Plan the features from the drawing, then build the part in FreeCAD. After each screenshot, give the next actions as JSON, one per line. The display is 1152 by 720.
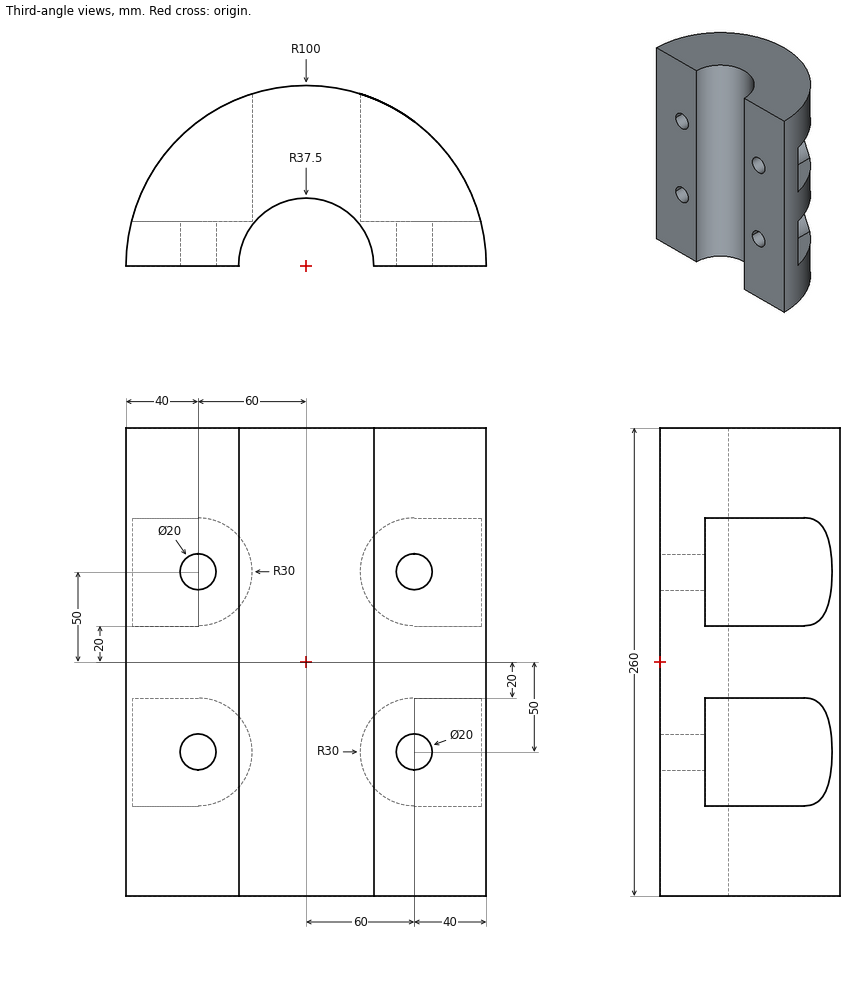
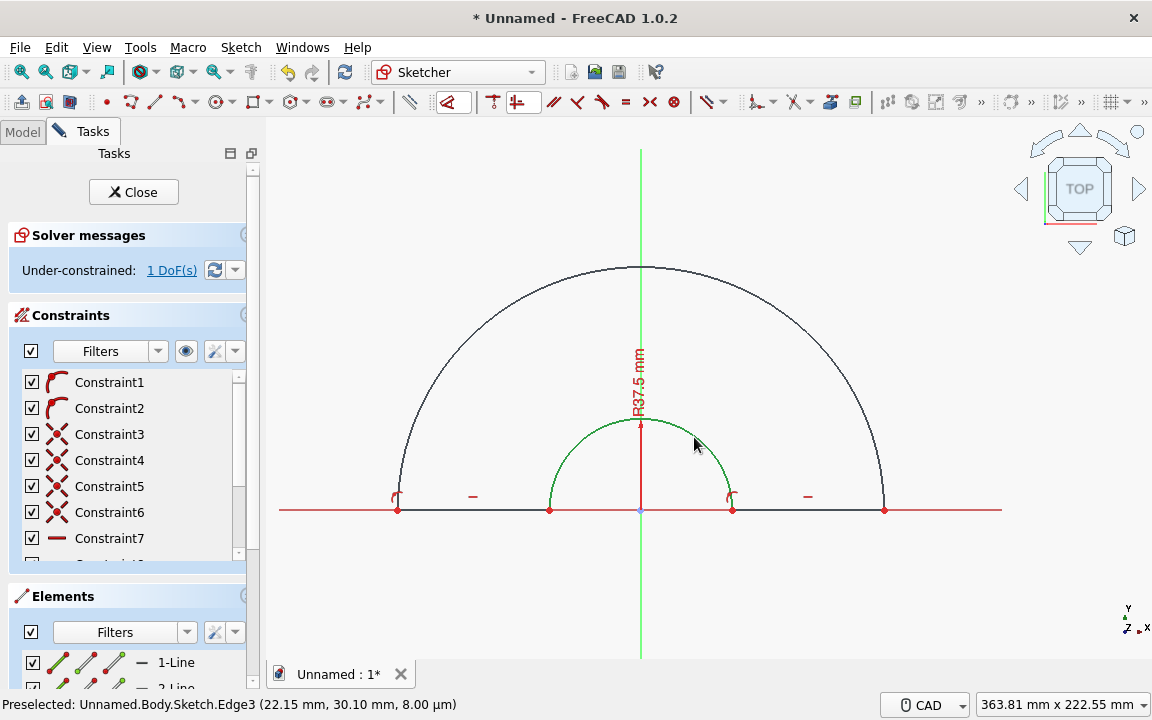
{"action": "left_click", "coordinate": [784, 313]}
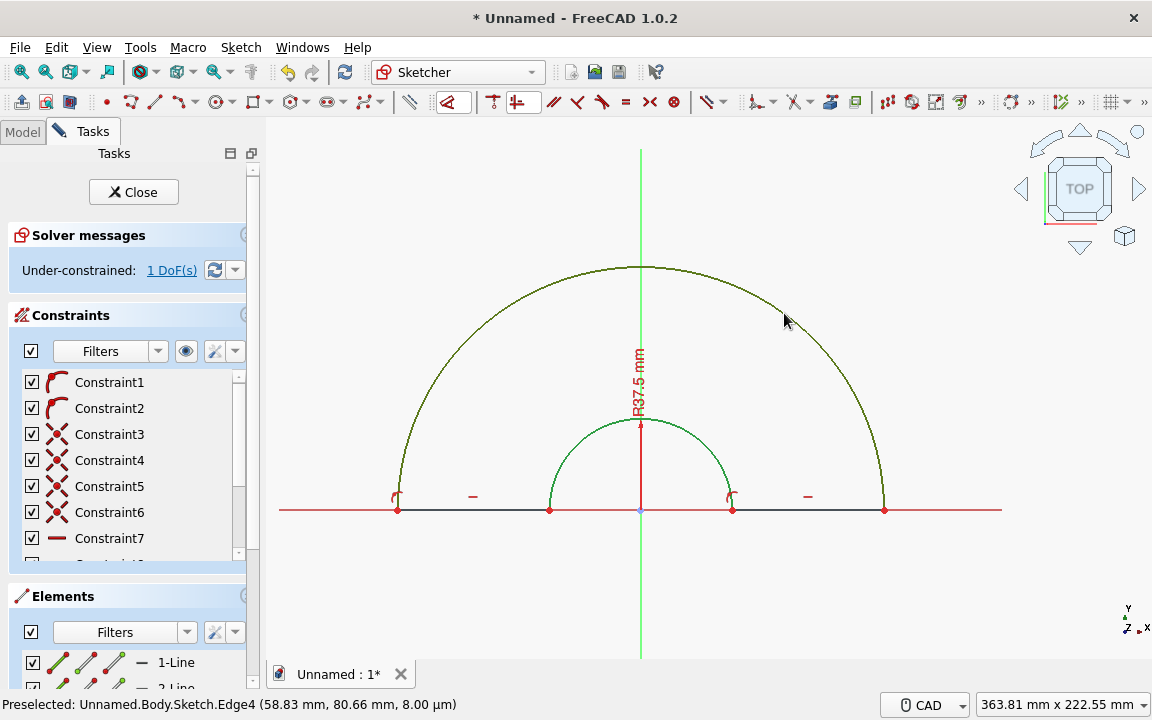
{"action": "key", "text": "k r"}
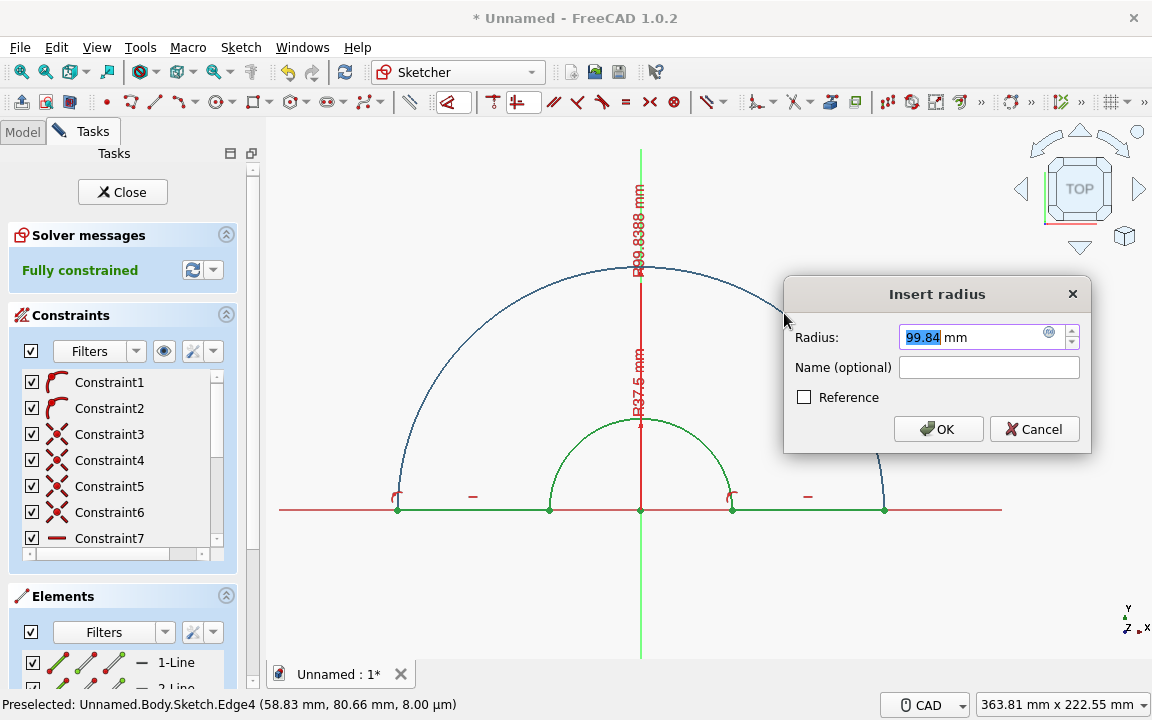
{"action": "type", "text": "100"}
{"action": "key", "text": "Return"}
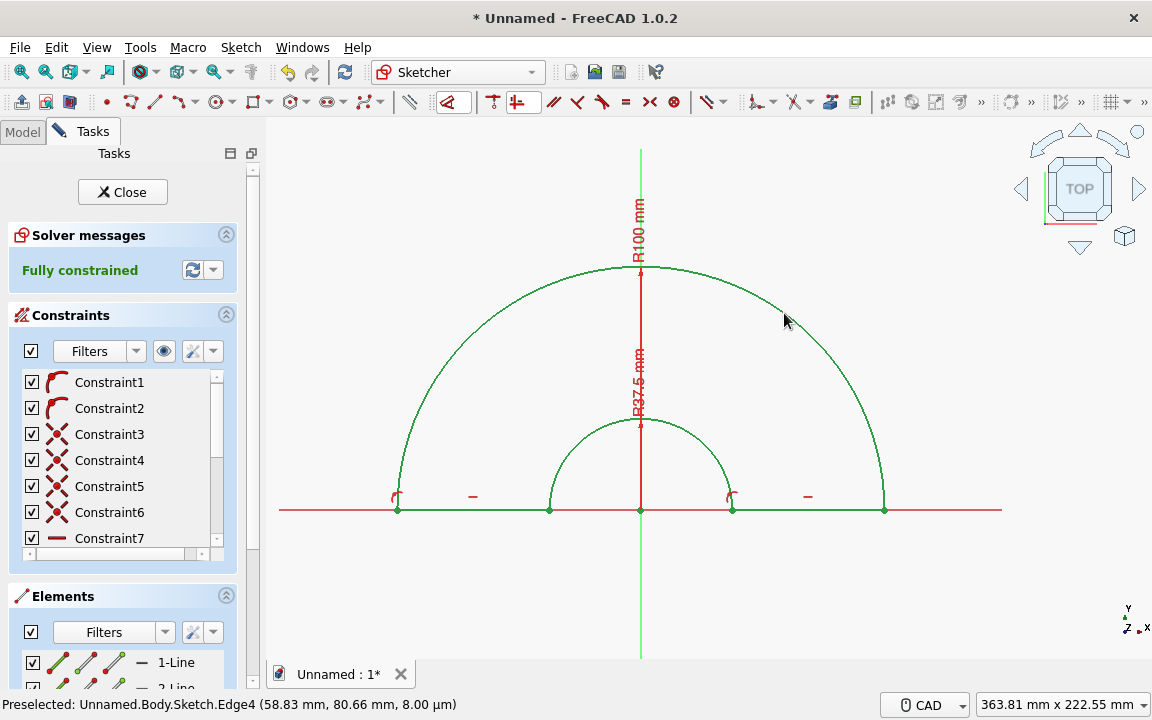
{"action": "left_click", "coordinate": [123, 192]}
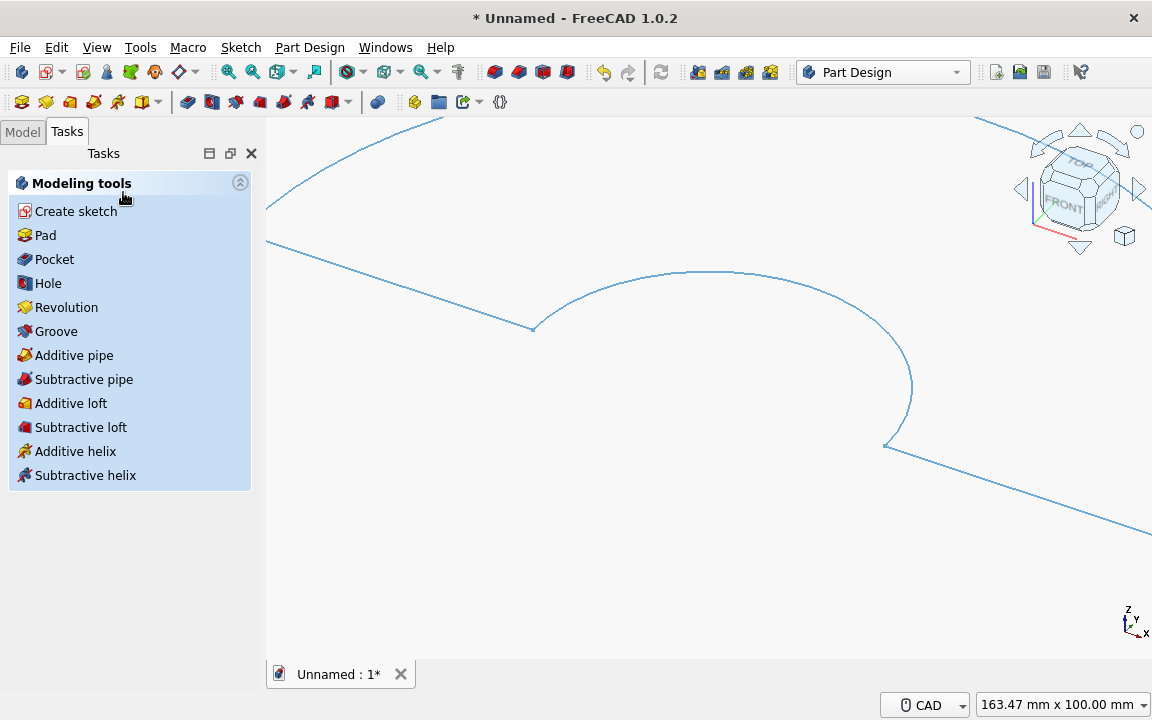
{"action": "left_click", "coordinate": [22, 102]}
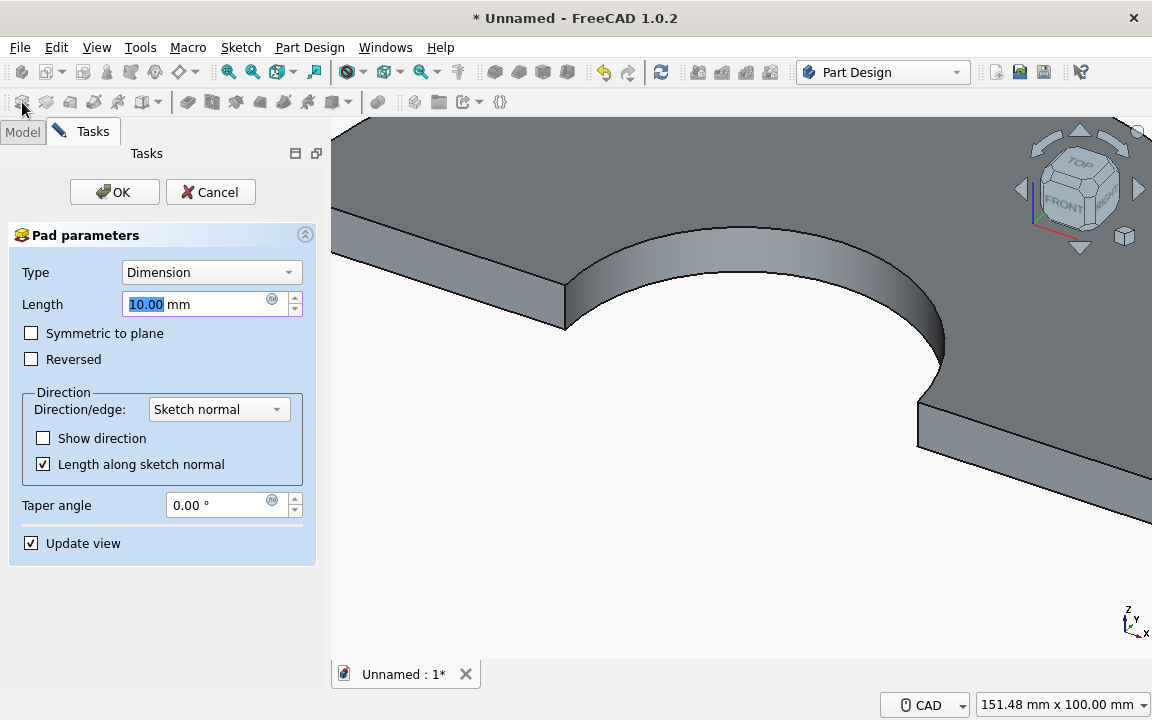
{"action": "type", "text": "260"}
{"action": "key", "text": "Tab"}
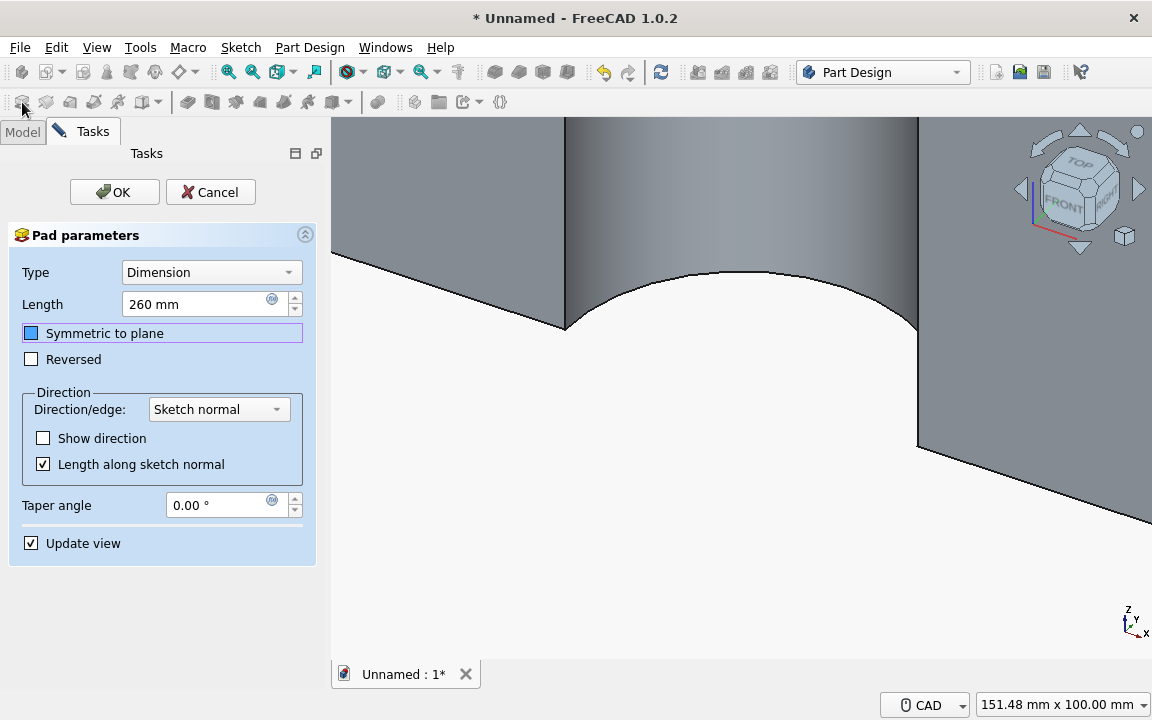
{"action": "left_click", "coordinate": [30, 333]}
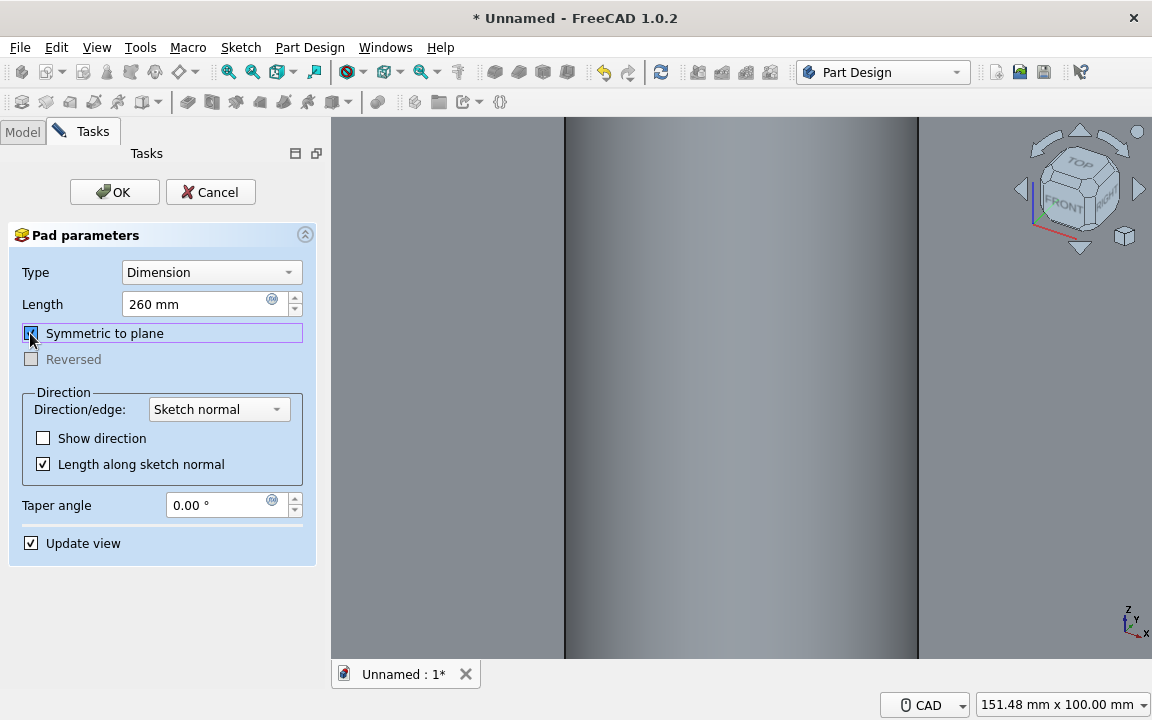
{"action": "left_click", "coordinate": [115, 192]}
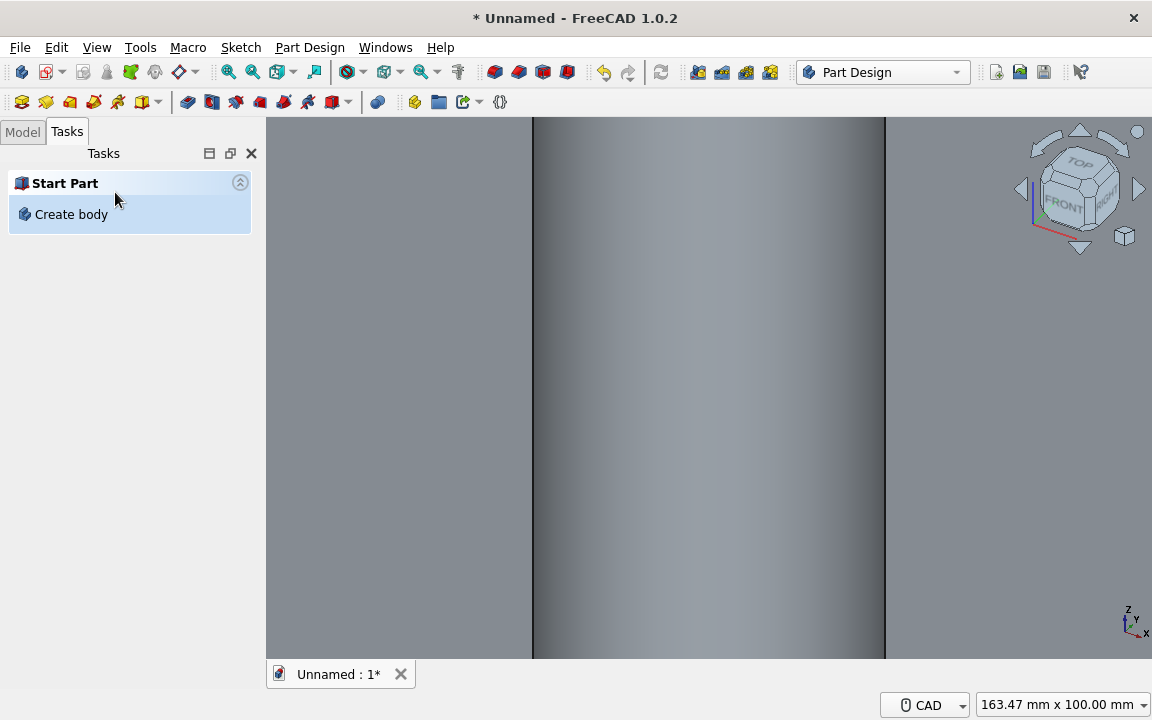
{"action": "left_click", "coordinate": [230, 72]}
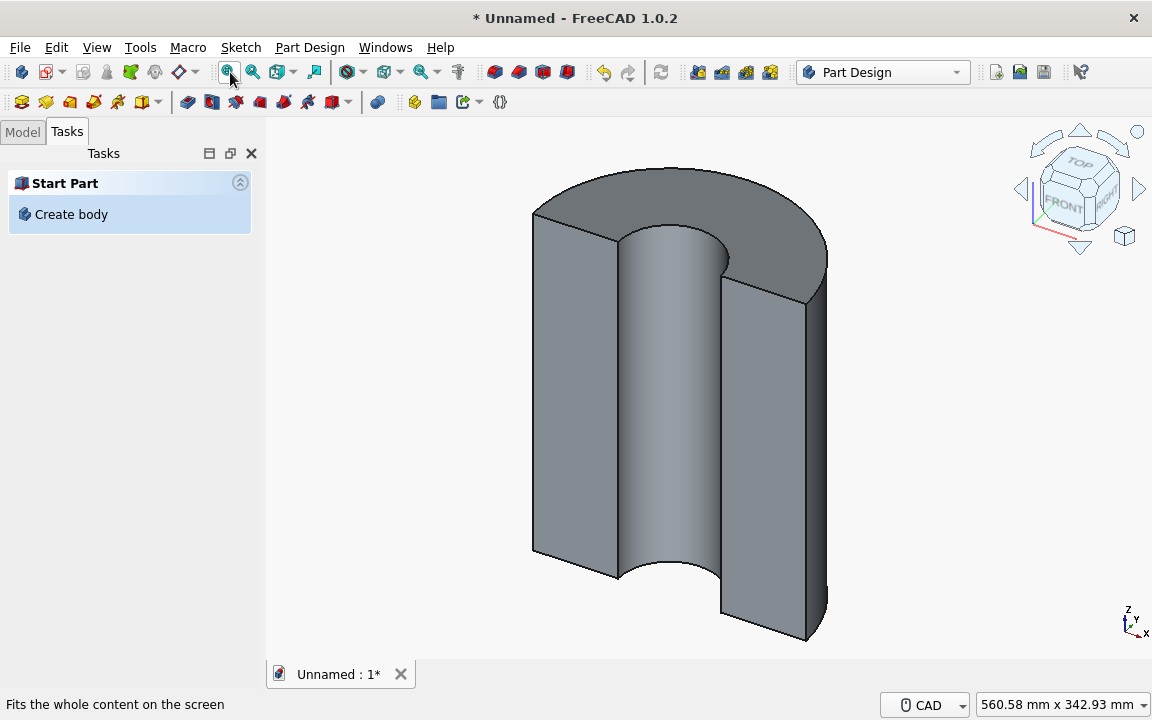
{"action": "left_click", "coordinate": [23, 131]}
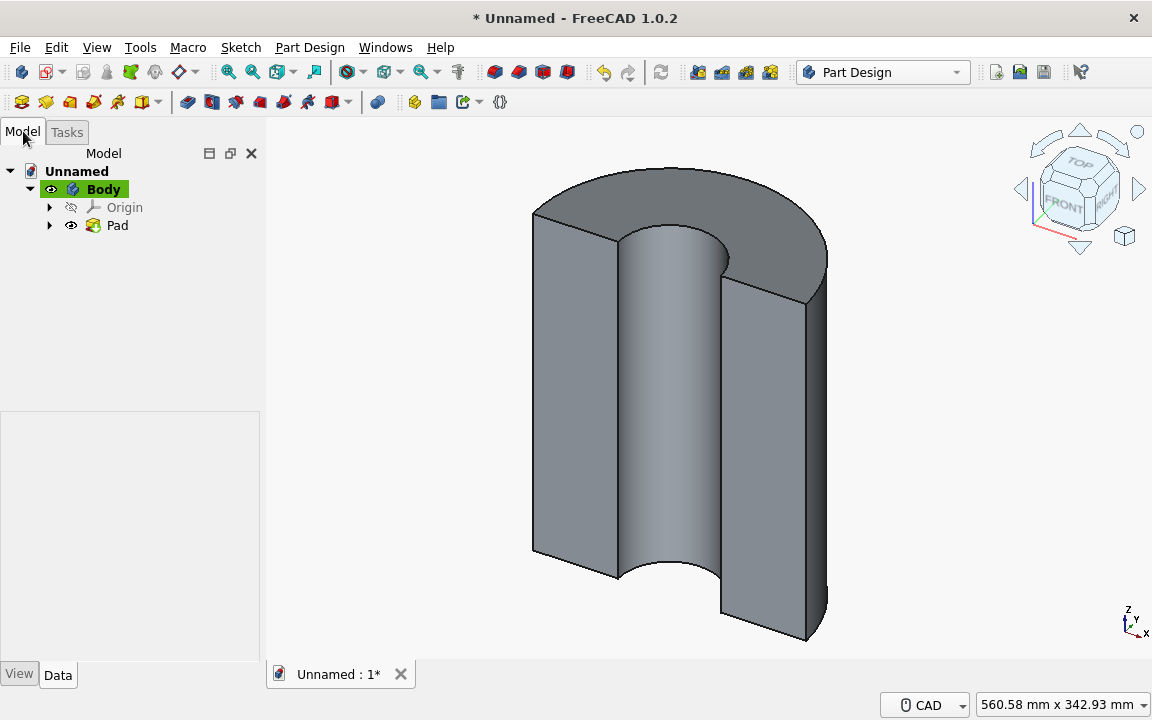
{"action": "left_click", "coordinate": [50, 207]}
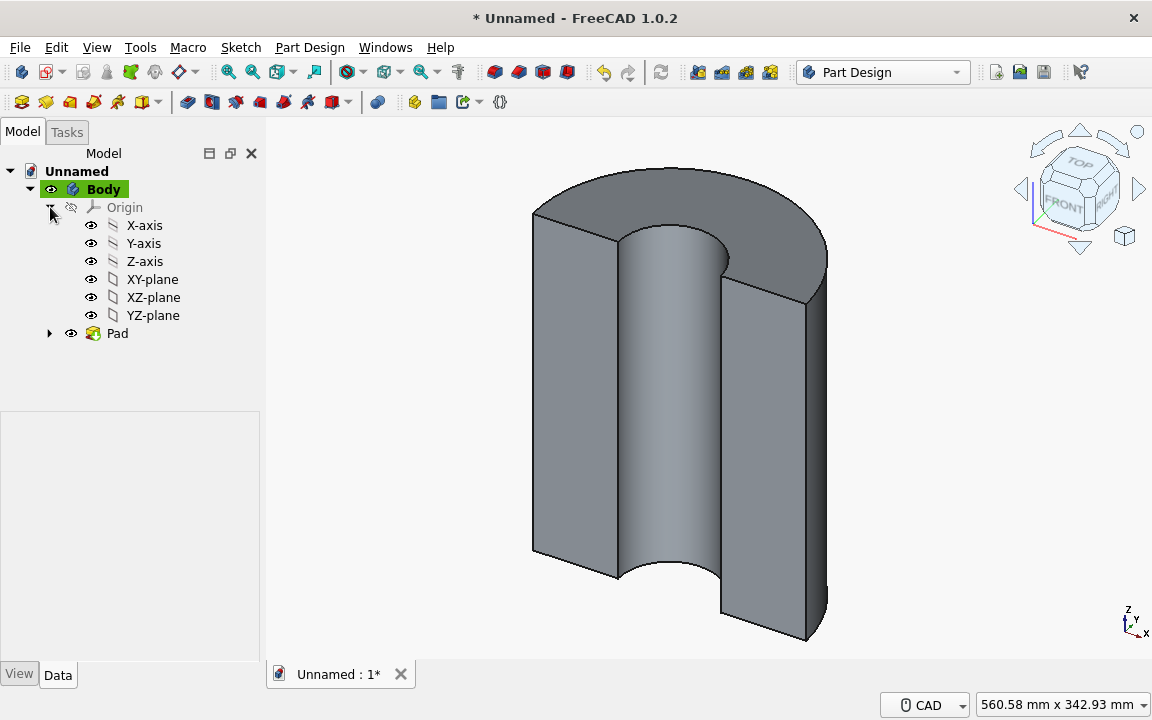
{"action": "left_click", "coordinate": [136, 297]}